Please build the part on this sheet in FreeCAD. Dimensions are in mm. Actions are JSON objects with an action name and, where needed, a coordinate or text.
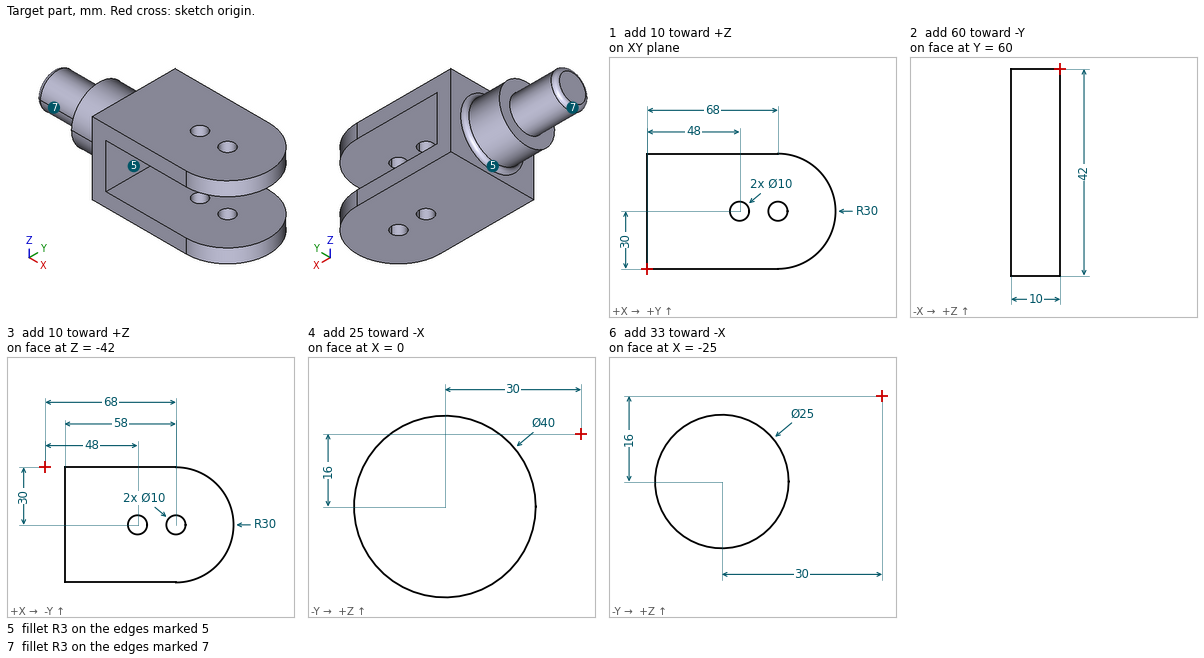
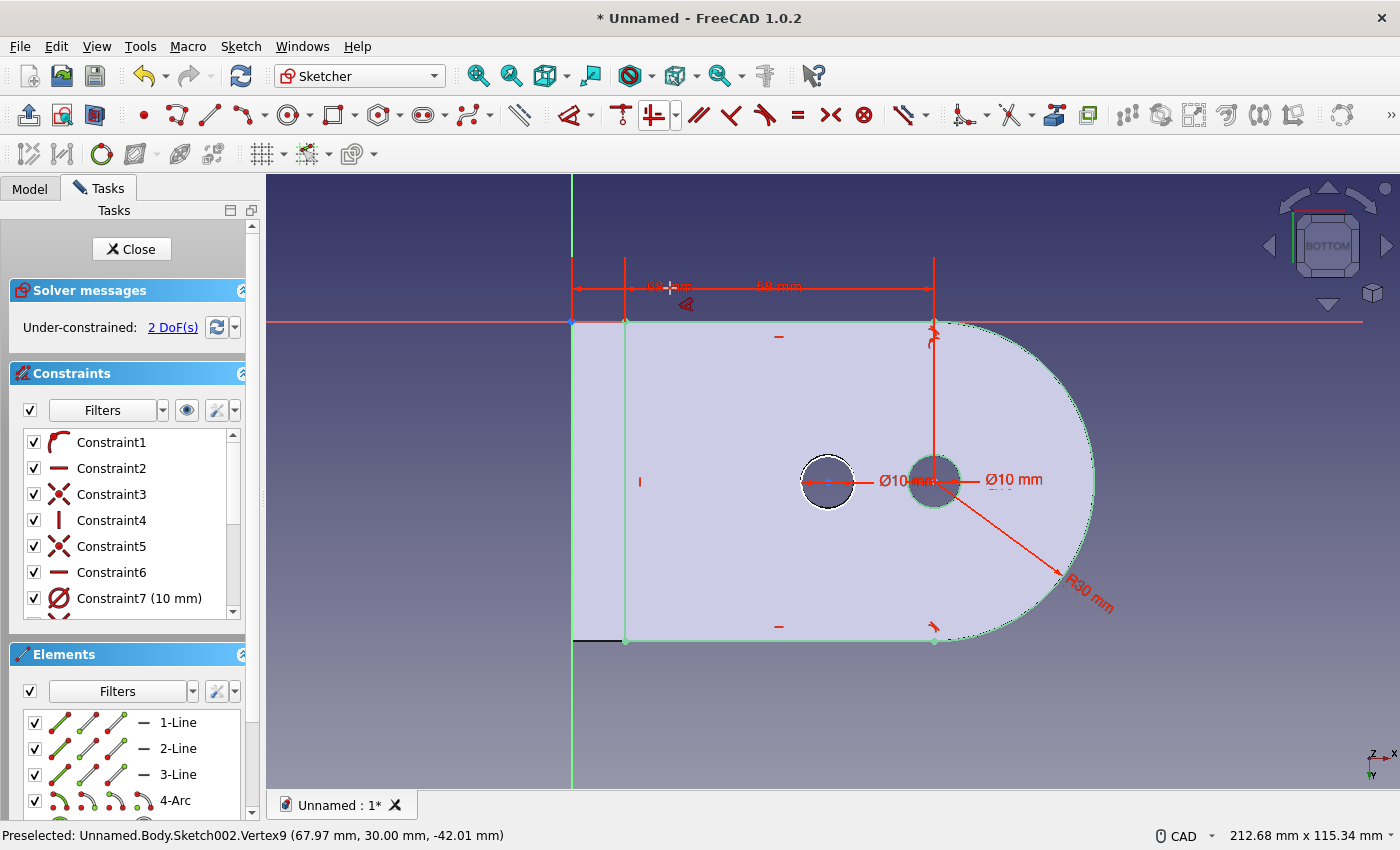
{"action": "left_click", "coordinate": [828, 483]}
{"action": "left_click", "coordinate": [700, 517]}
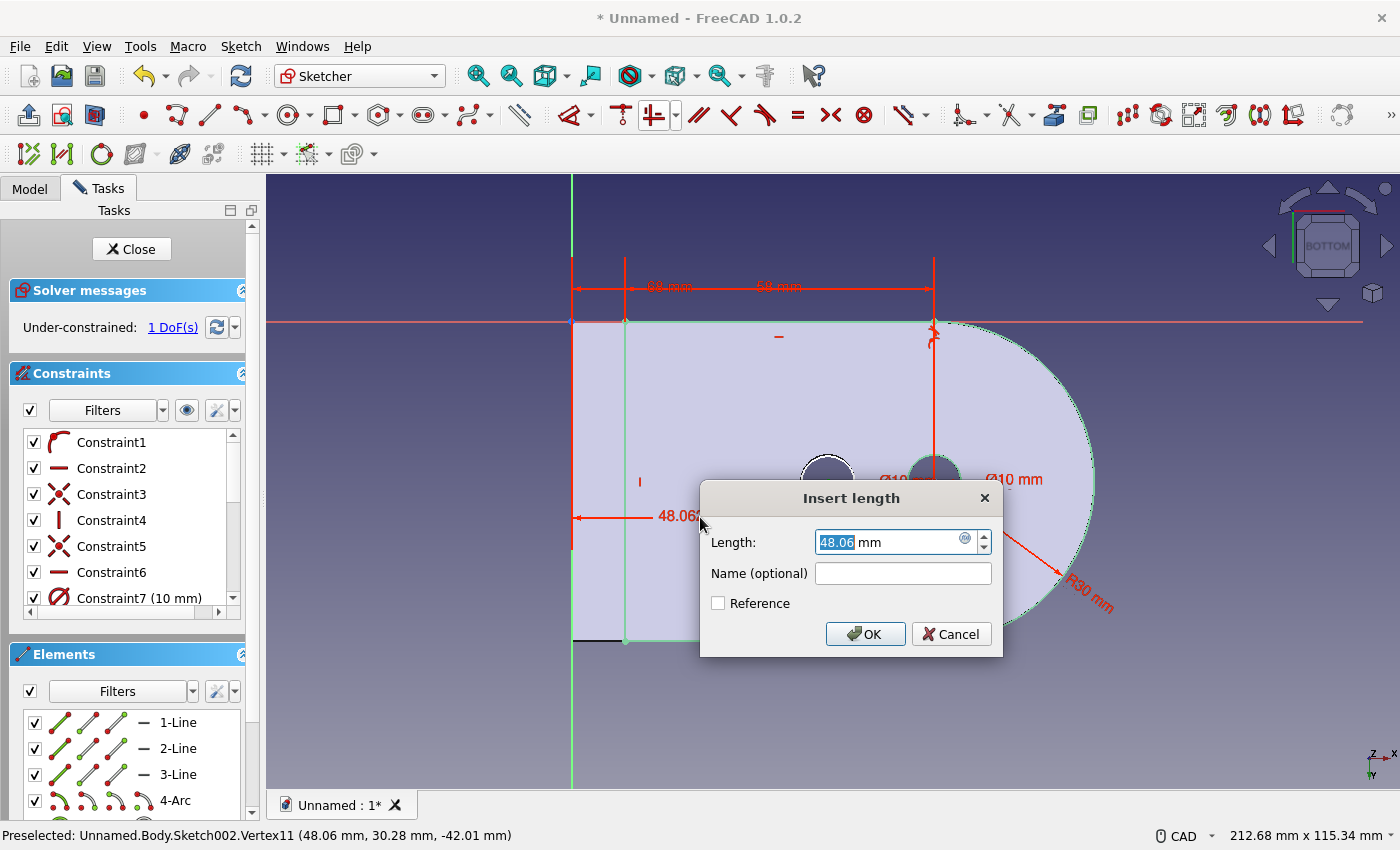
{"action": "type", "text": "48"}
{"action": "key", "text": "Return"}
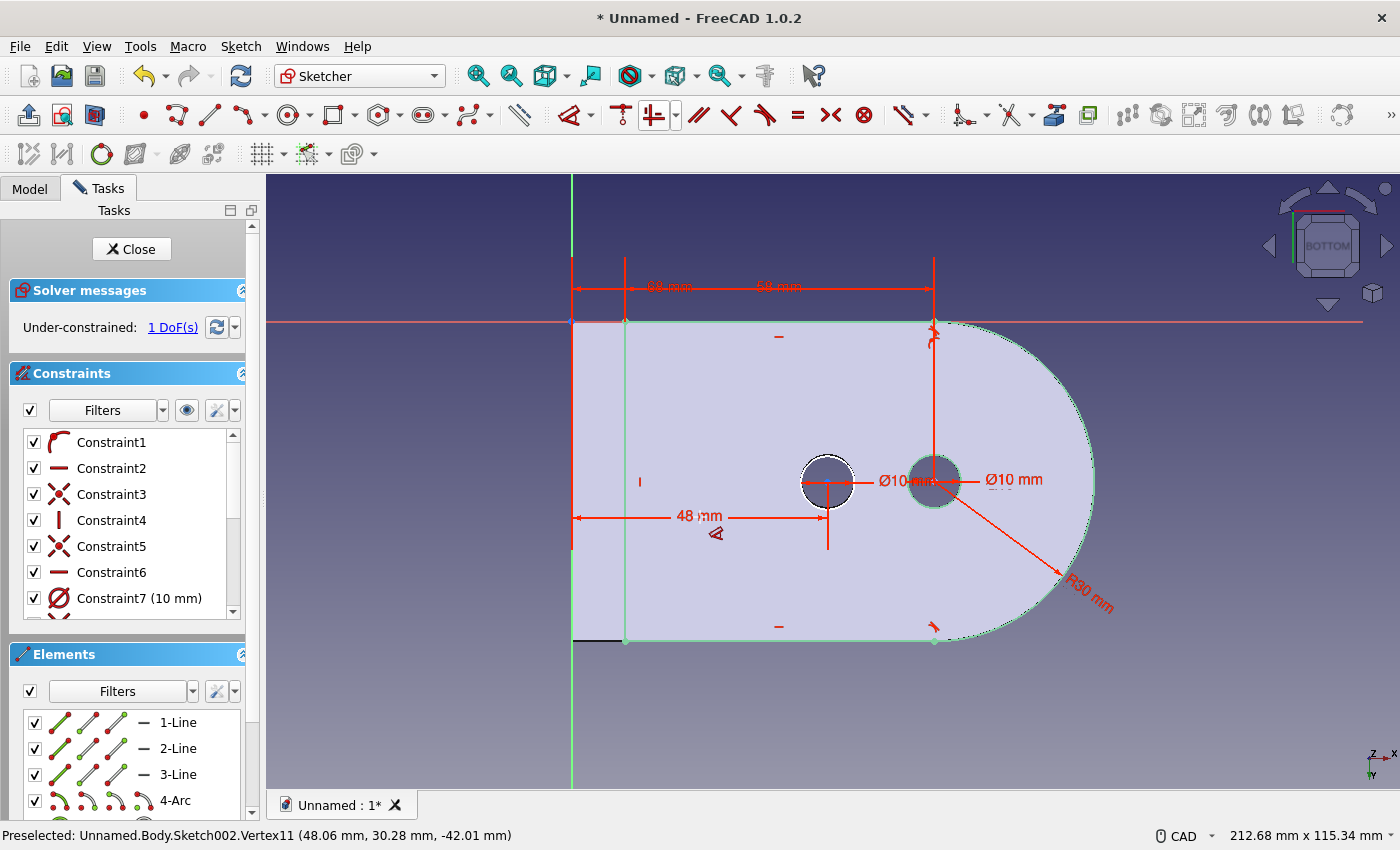
{"action": "left_click", "coordinate": [828, 483]}
{"action": "left_click", "coordinate": [538, 402]}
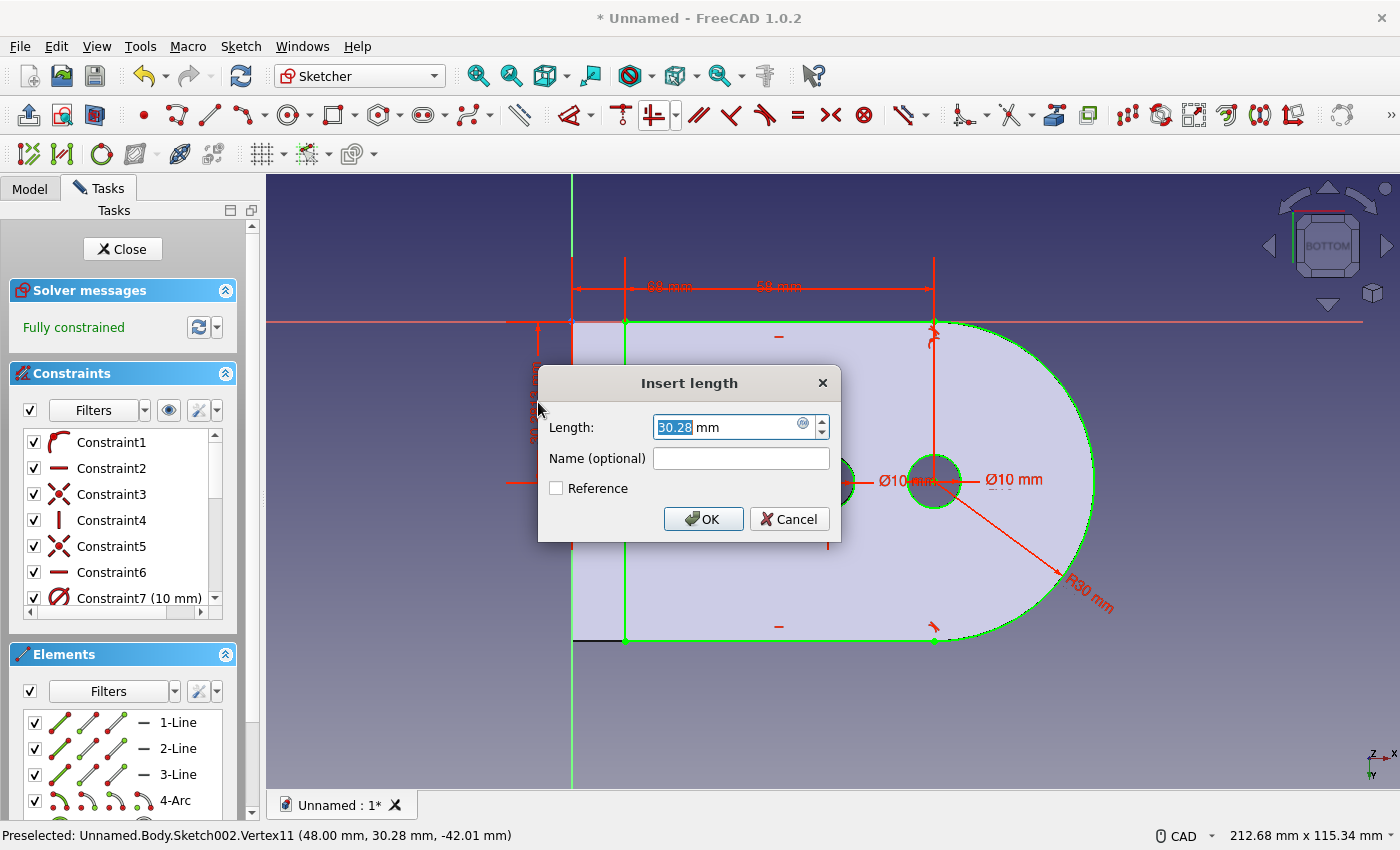
{"action": "type", "text": "30"}
{"action": "key", "text": "Return"}
{"action": "key", "text": "Escape"}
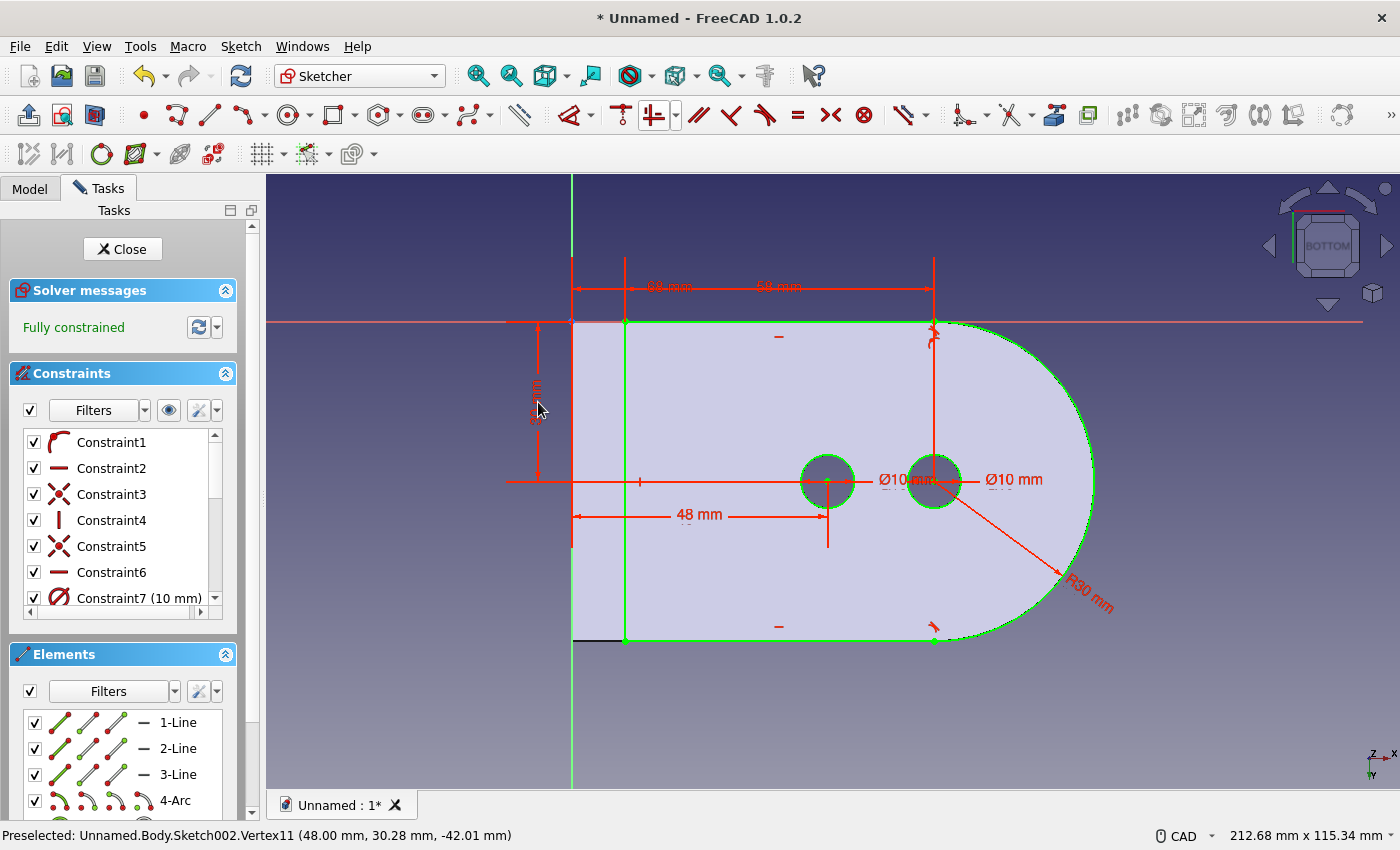
{"action": "left_click", "coordinate": [123, 249]}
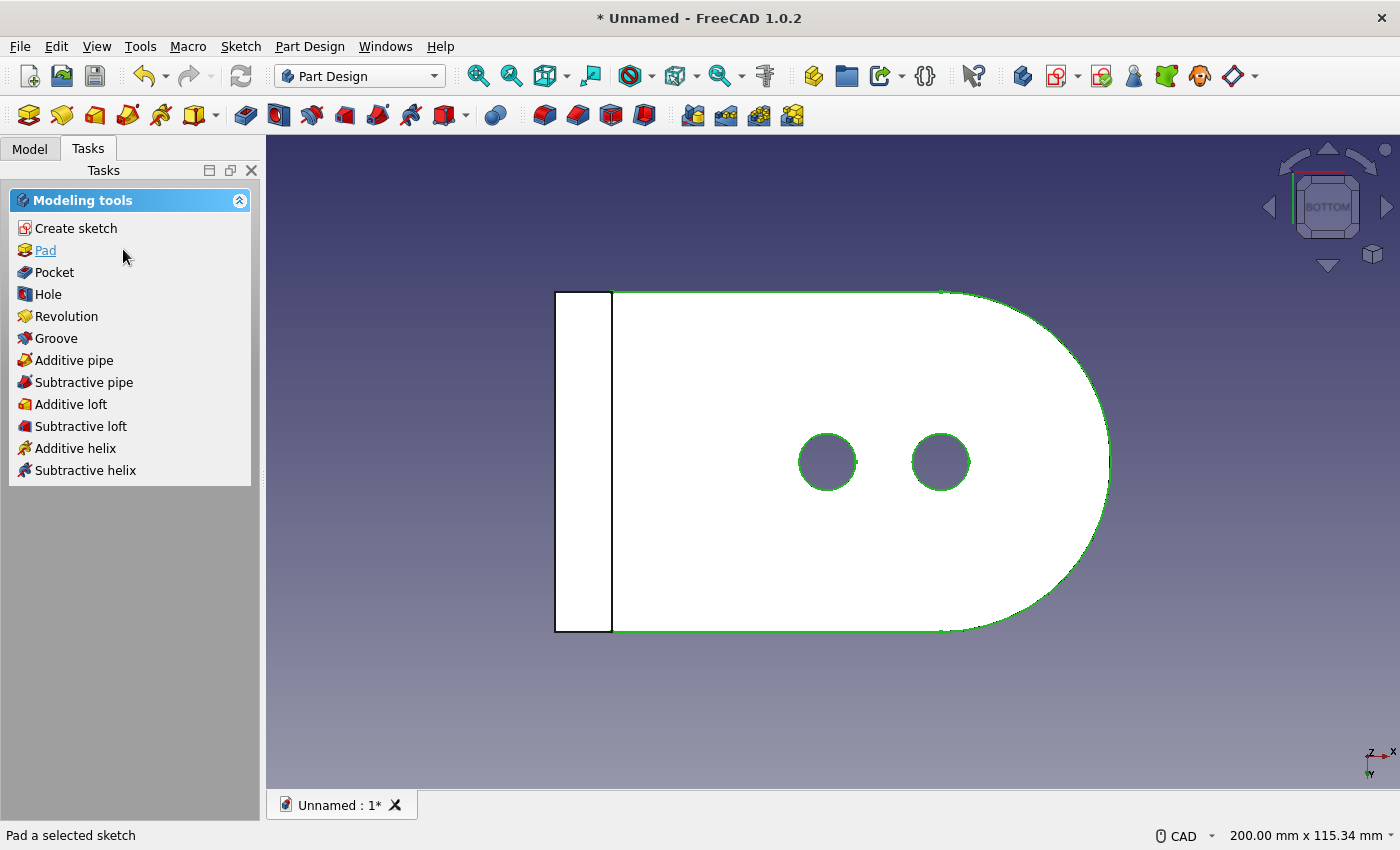
{"action": "left_click", "coordinate": [29, 116]}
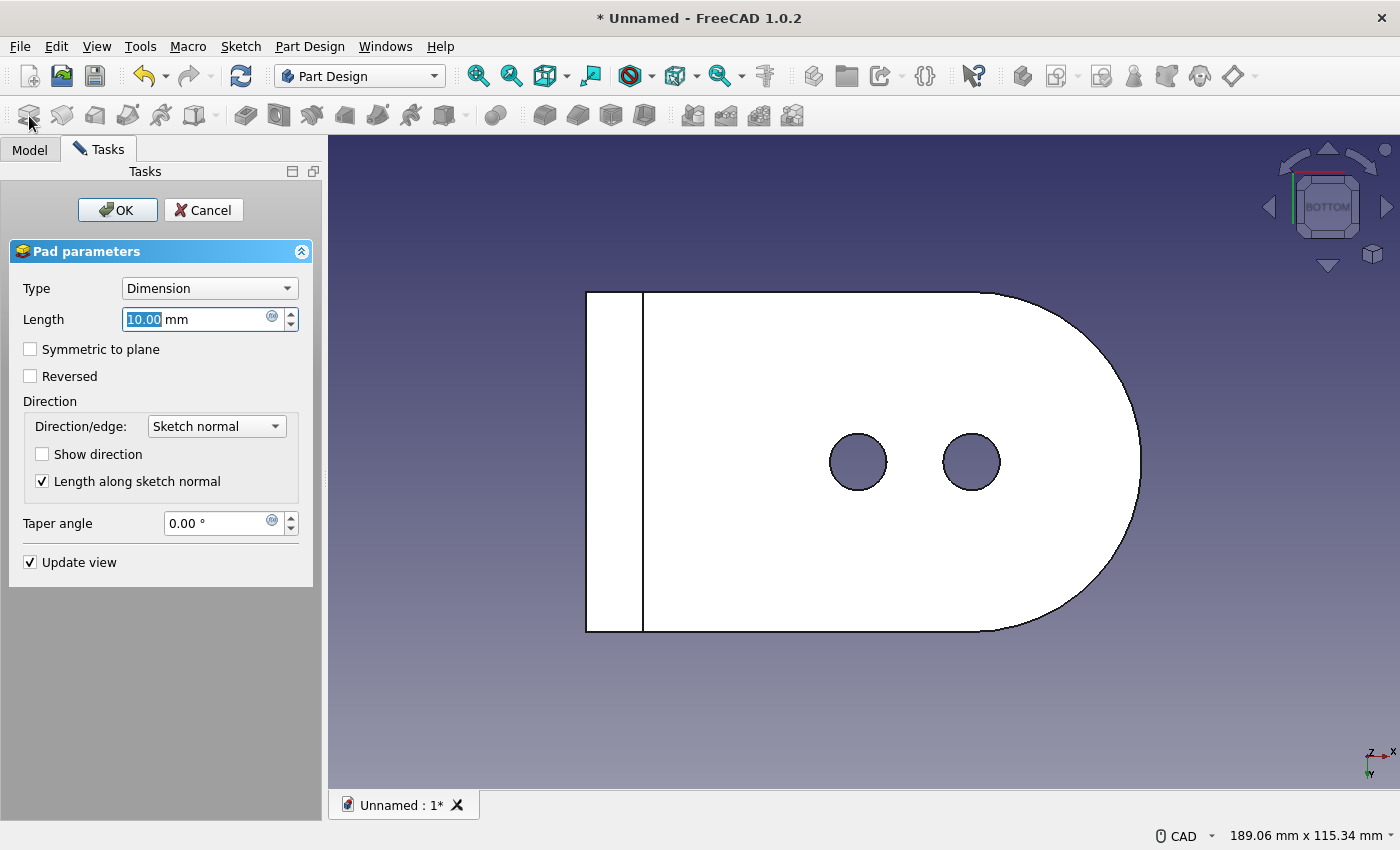
{"action": "type", "text": "10"}
{"action": "key", "text": "Tab"}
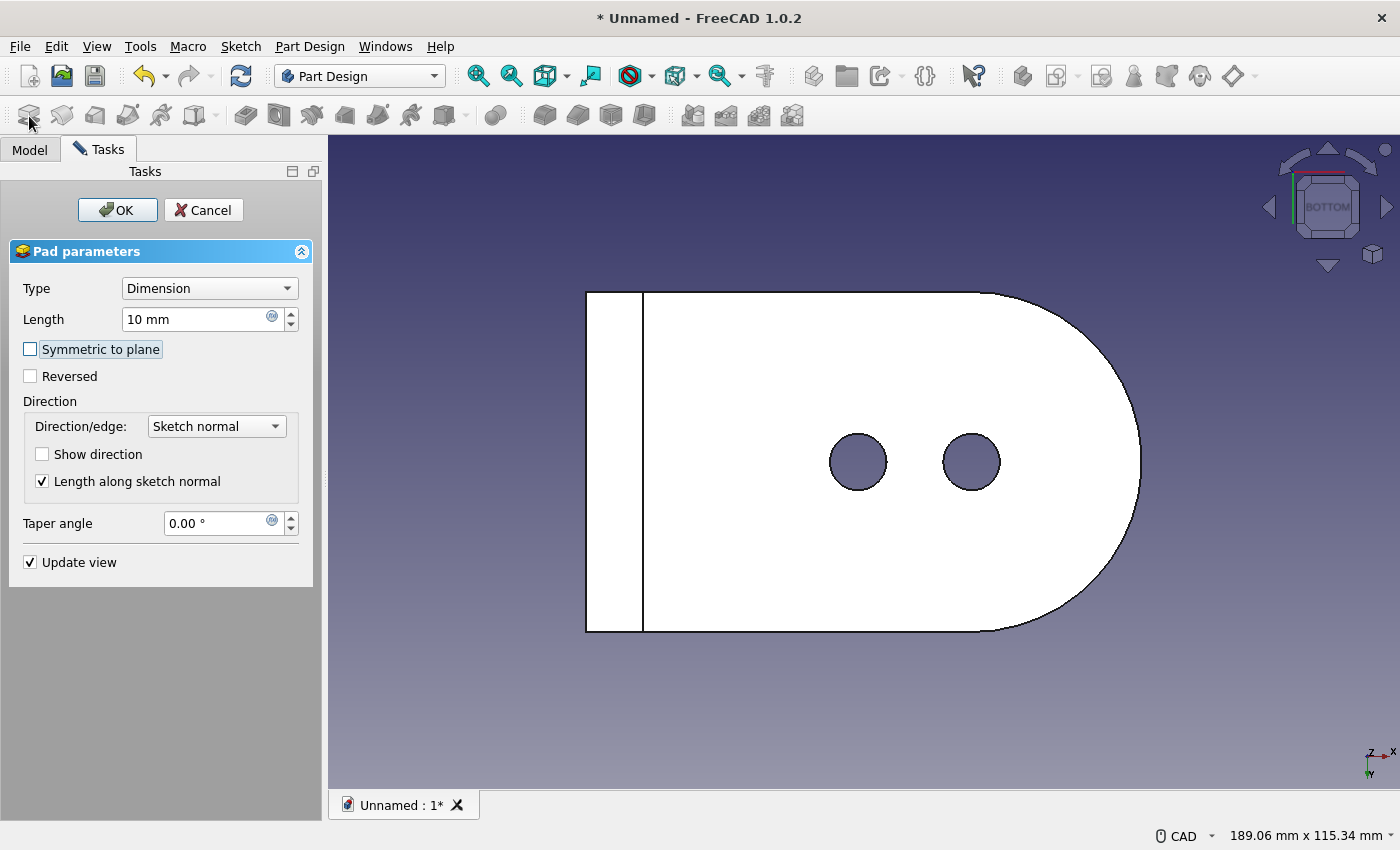
{"action": "left_click", "coordinate": [31, 376]}